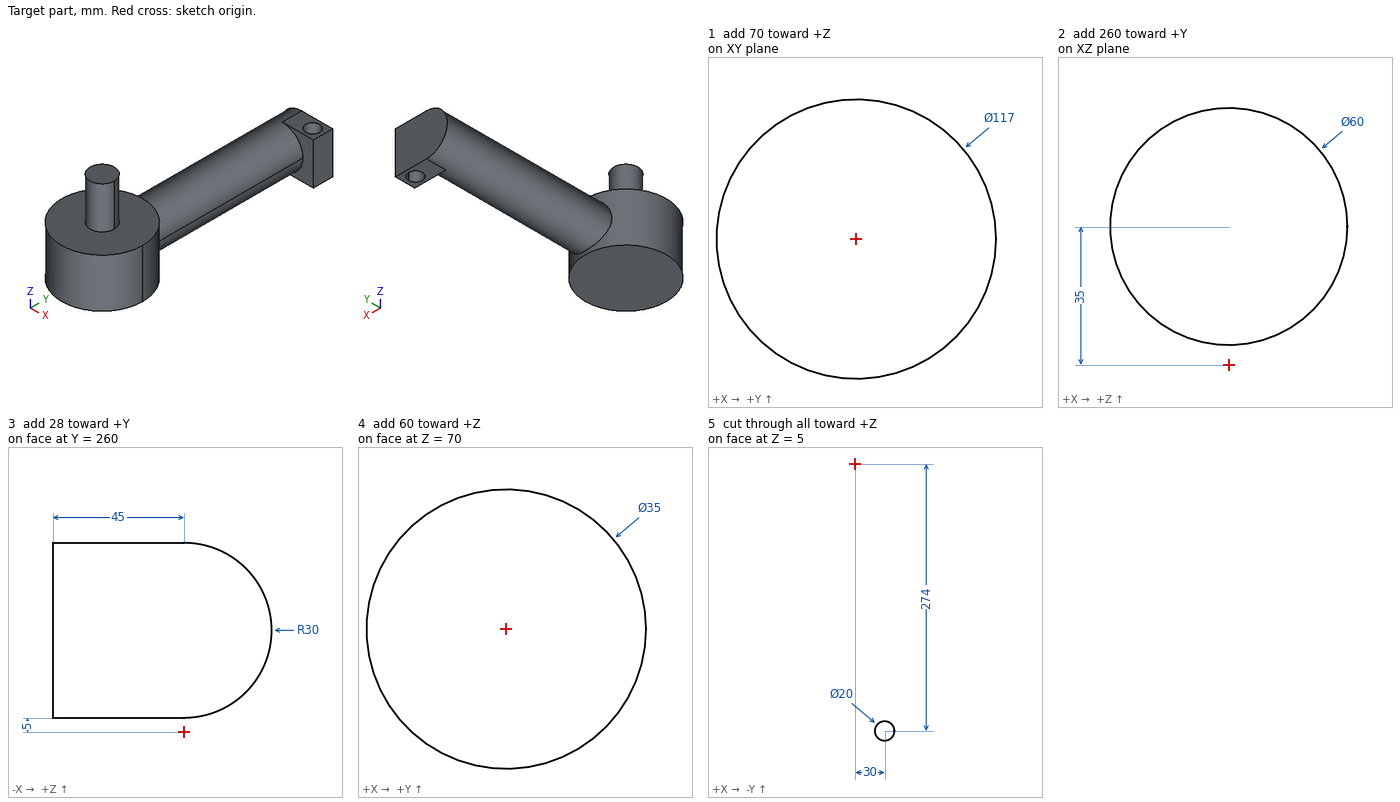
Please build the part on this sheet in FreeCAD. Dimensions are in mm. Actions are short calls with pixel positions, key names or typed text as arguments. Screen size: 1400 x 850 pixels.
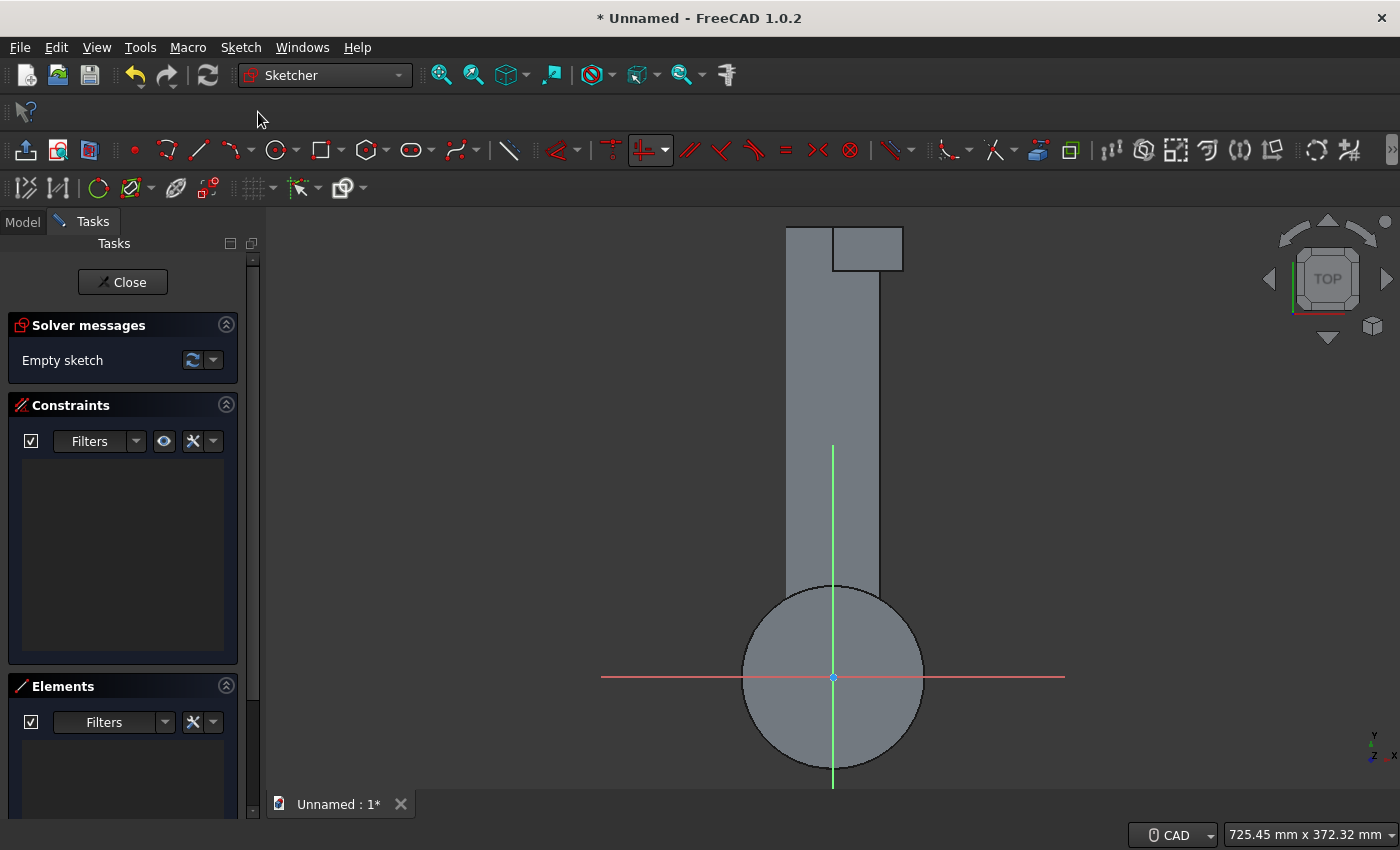
scroll(844, 705, up, 10)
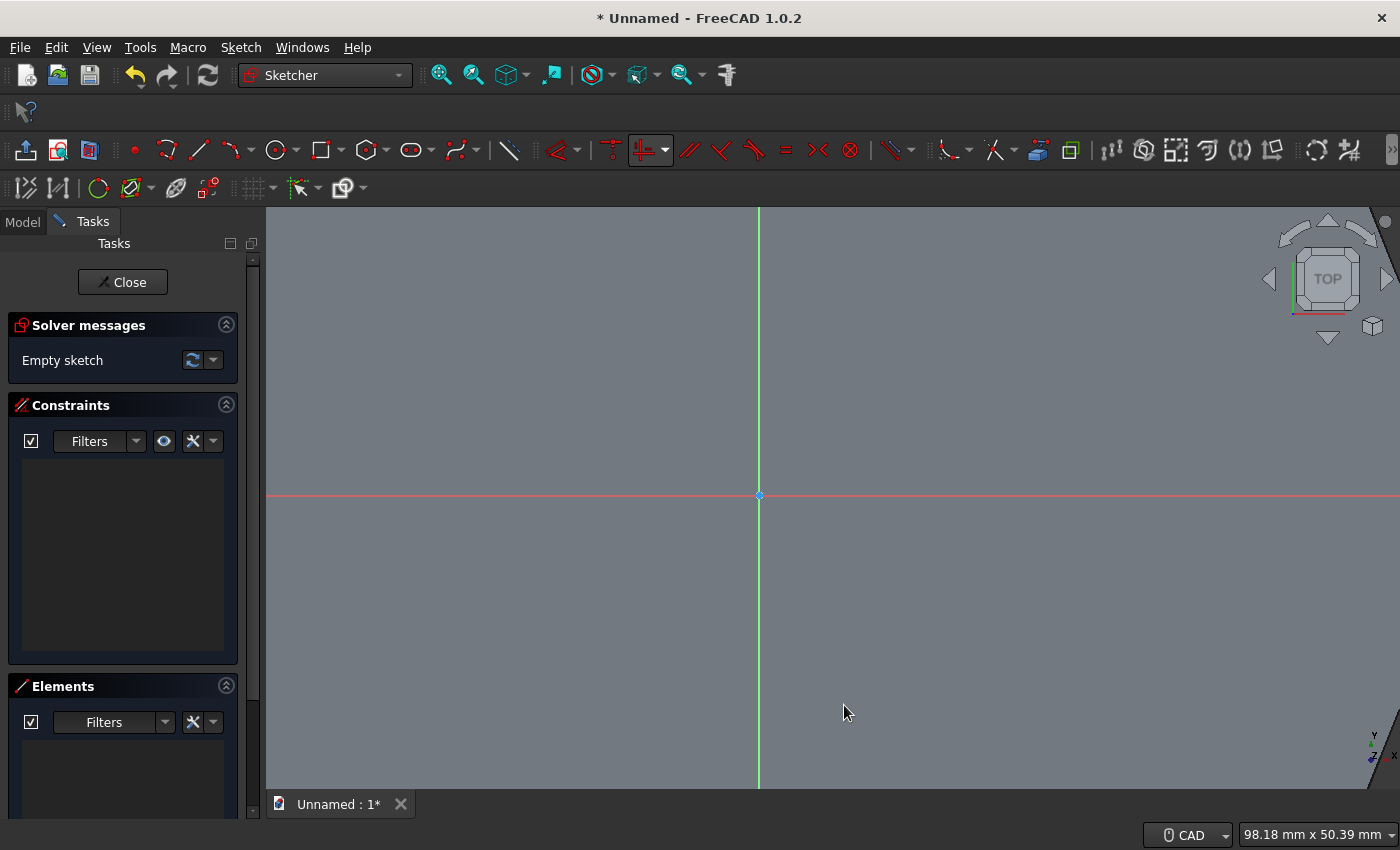
key(g)
key(c)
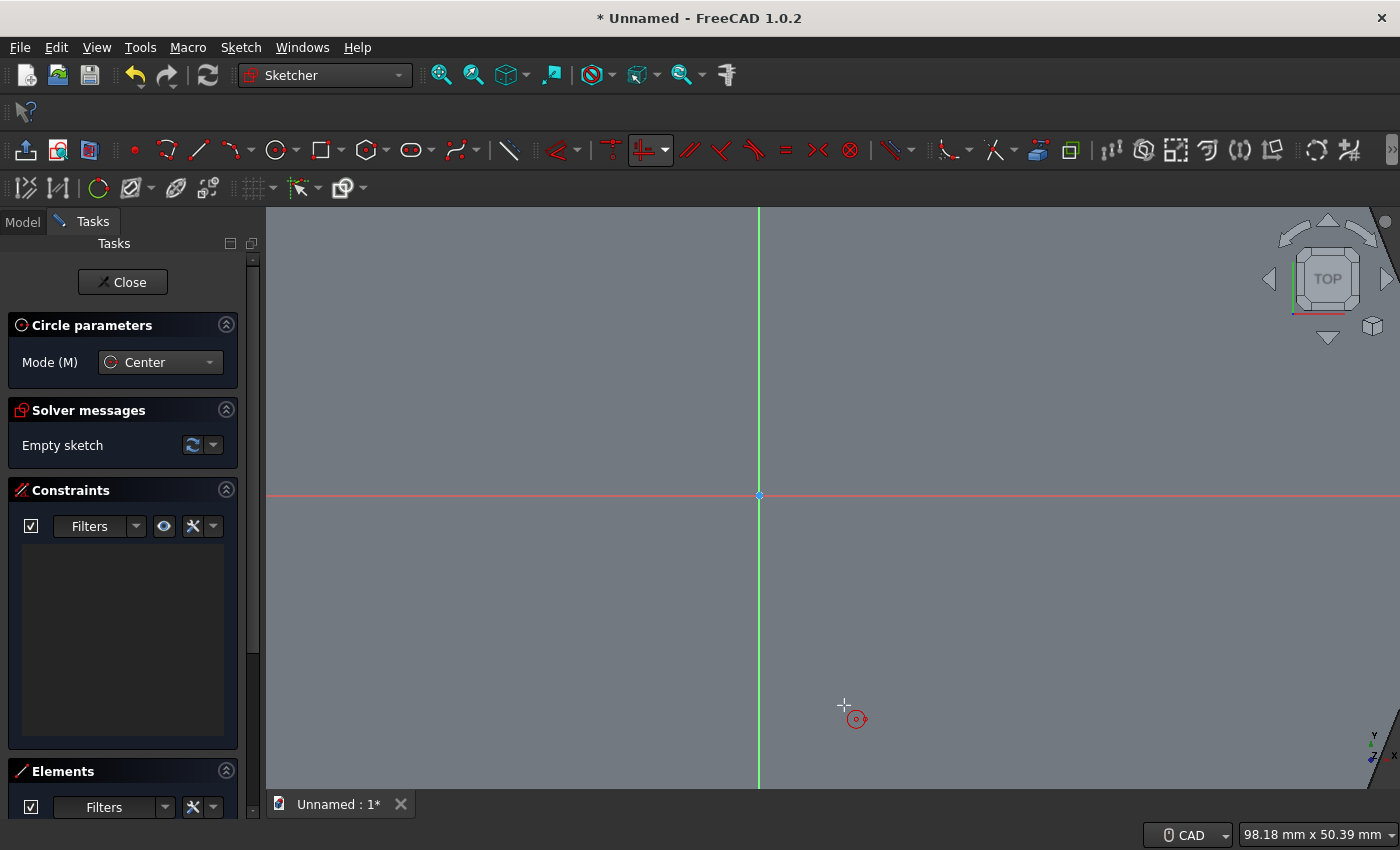
click(759, 496)
click(902, 353)
key(Escape)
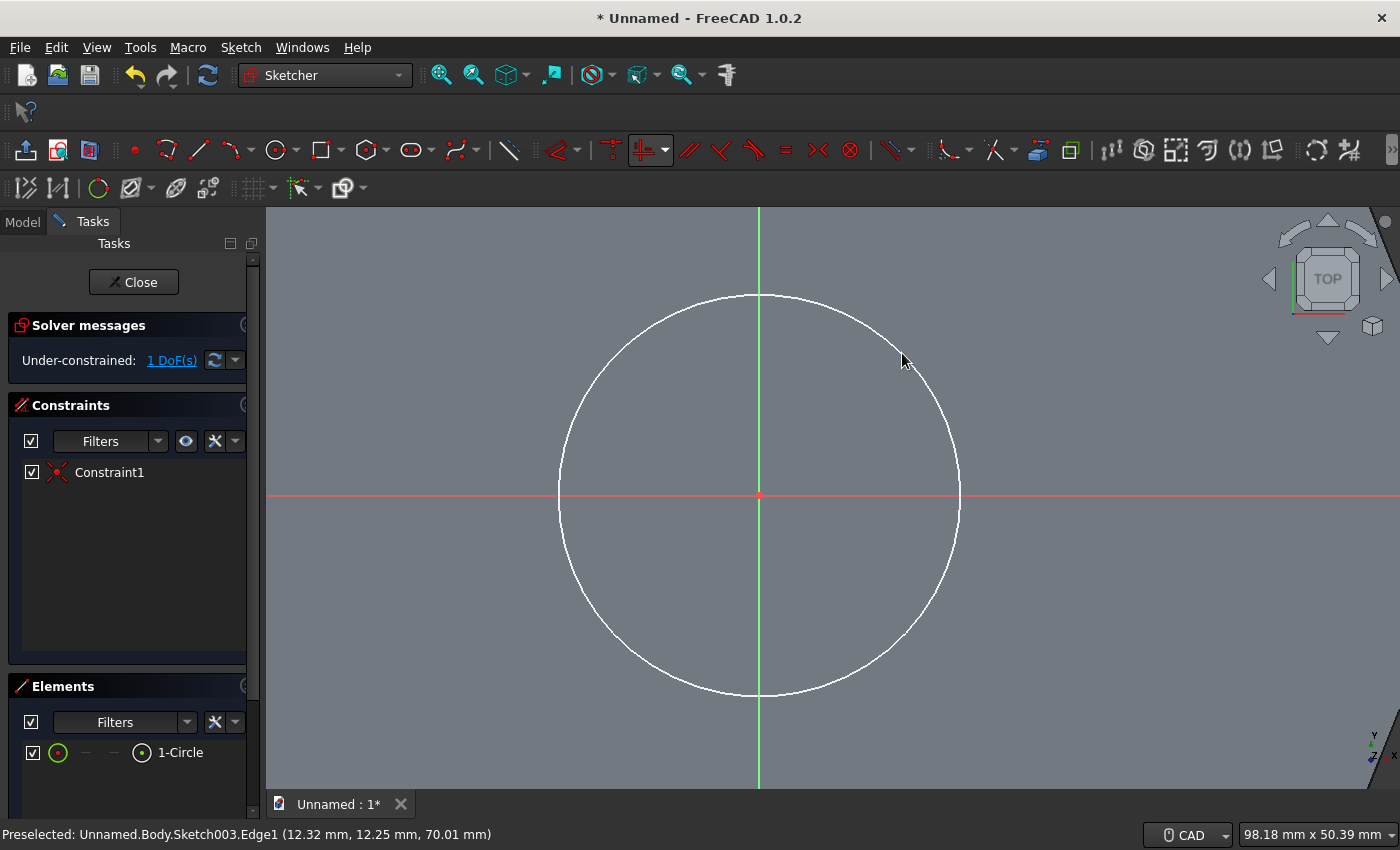
click(556, 150)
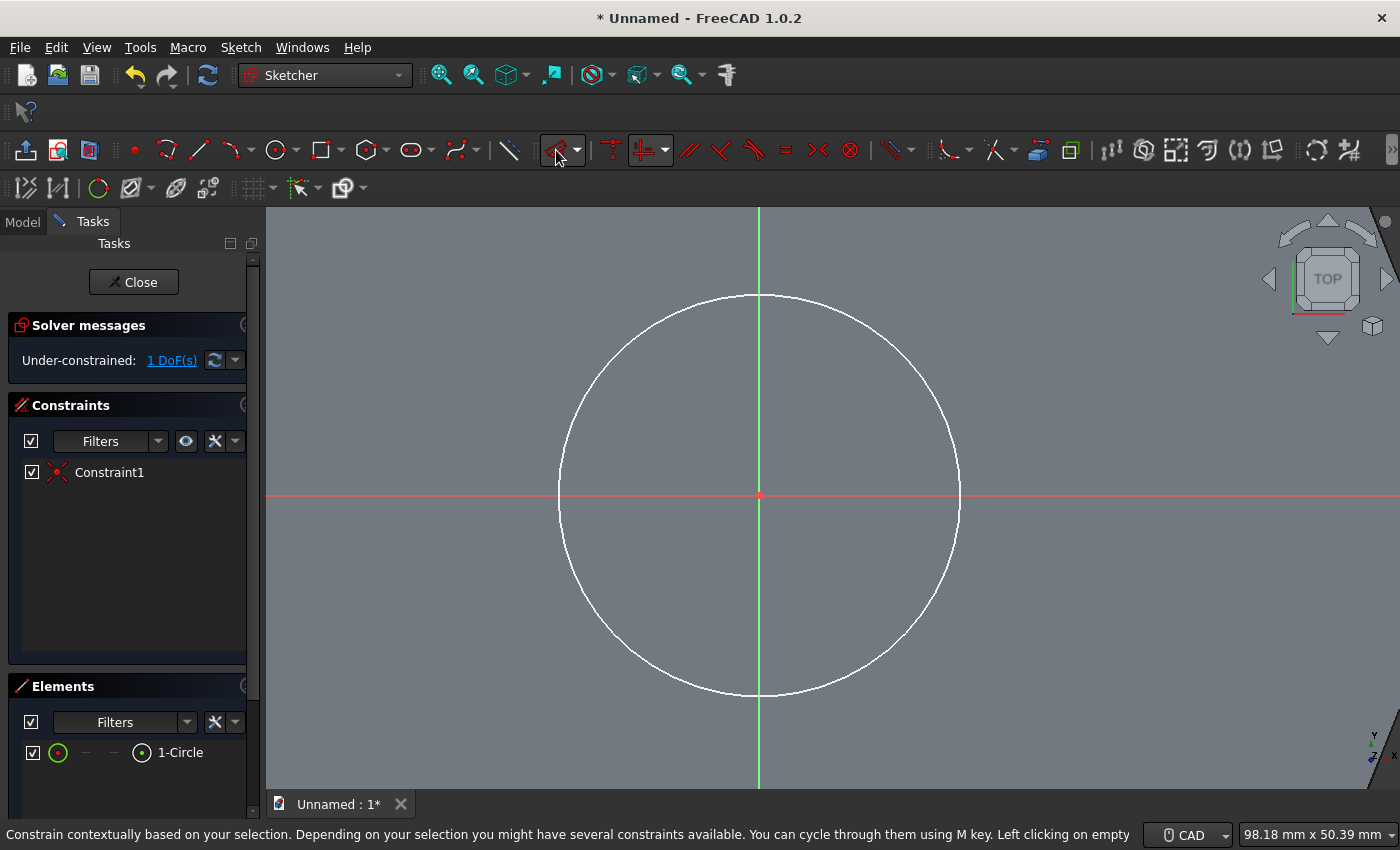
click(901, 353)
click(924, 330)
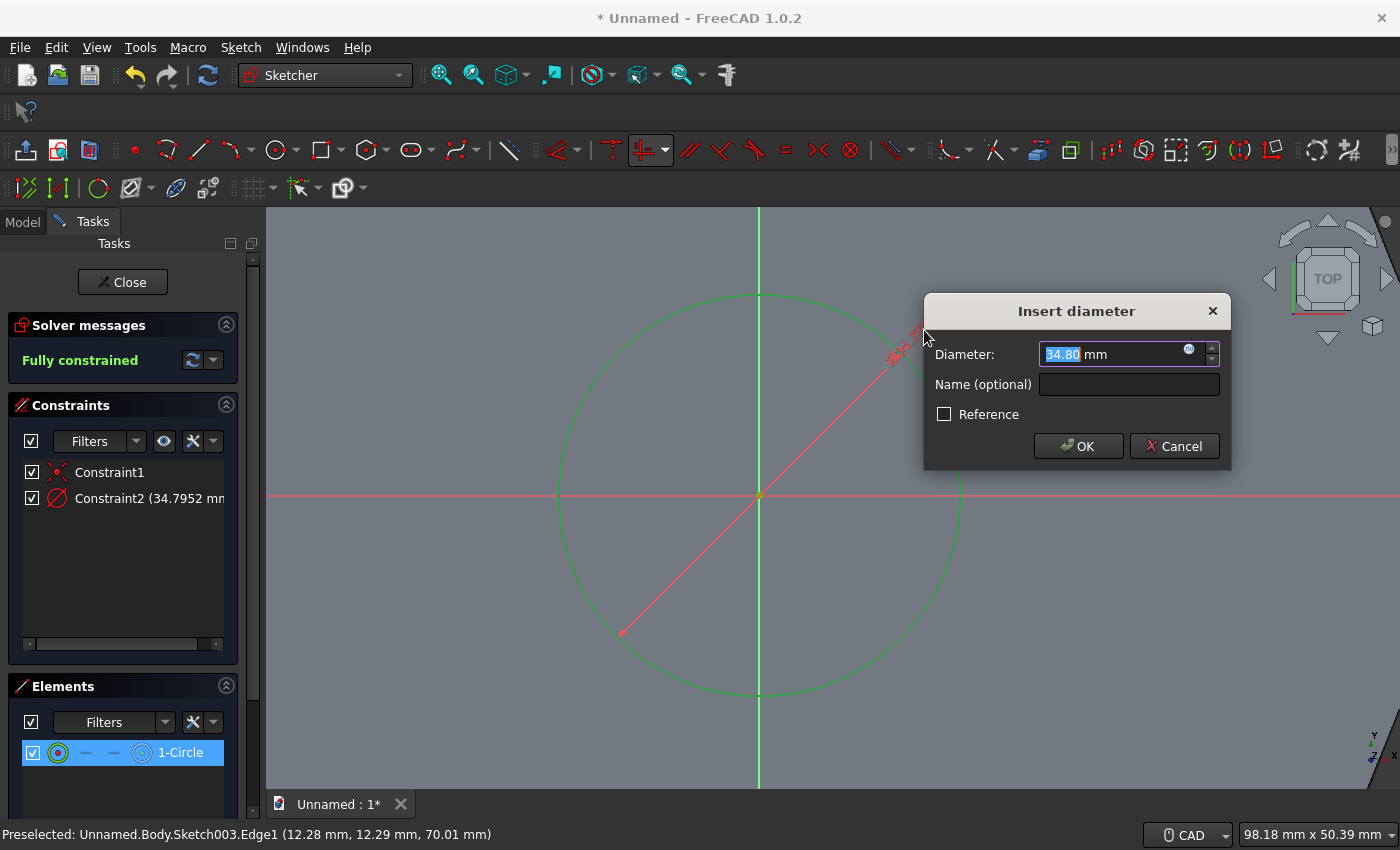
text(35)
key(Return)
key(Escape)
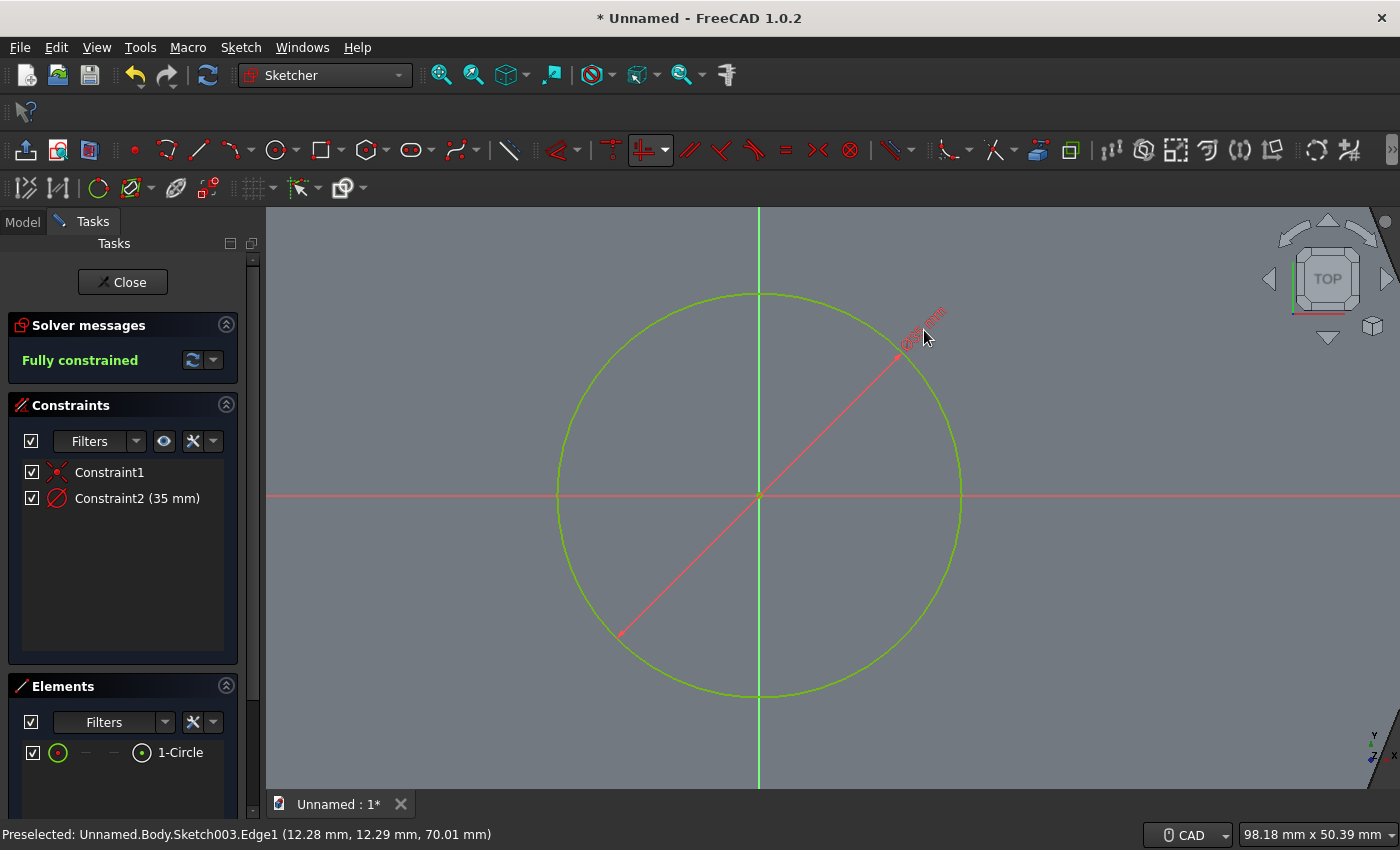
click(123, 282)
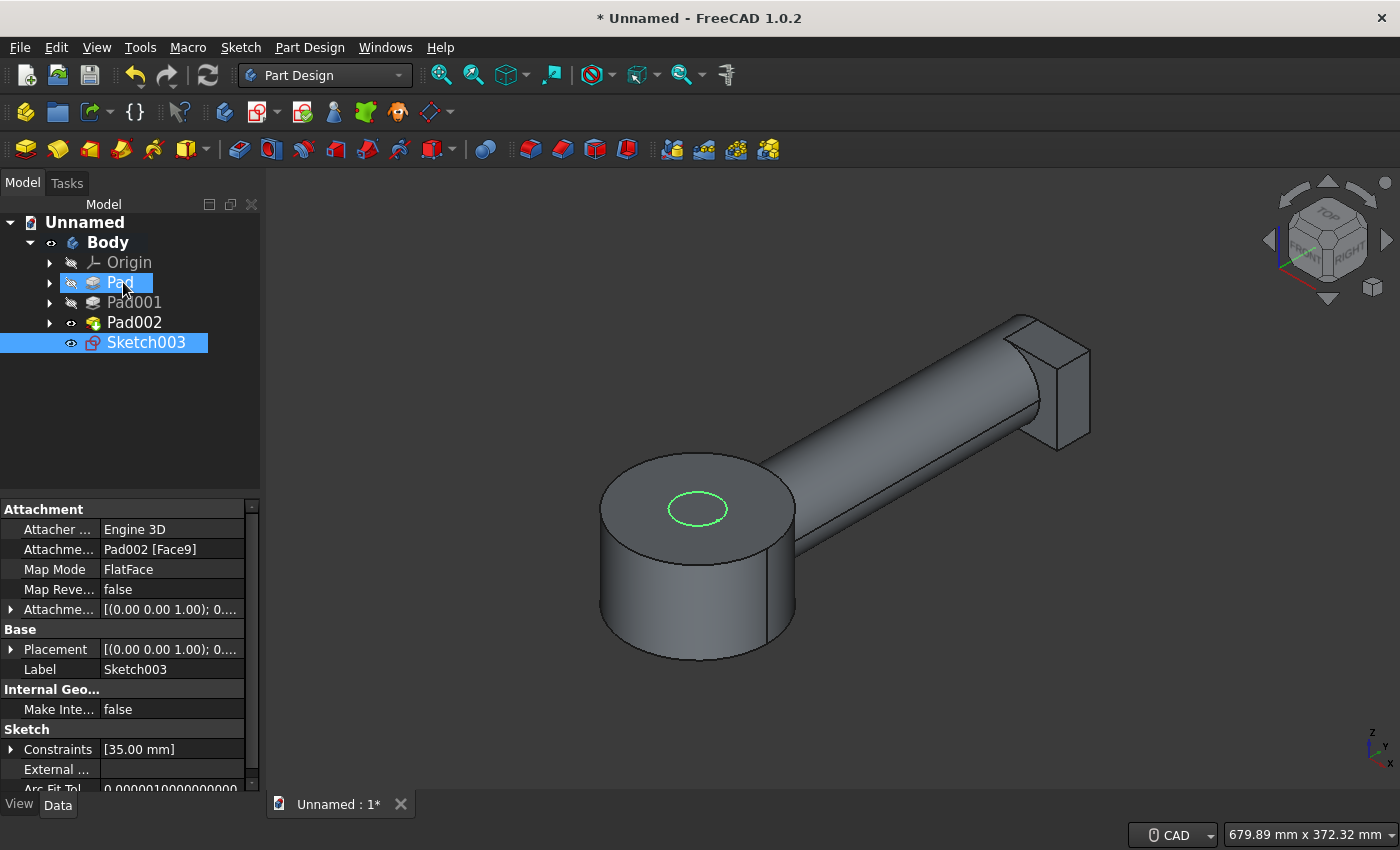
click(26, 150)